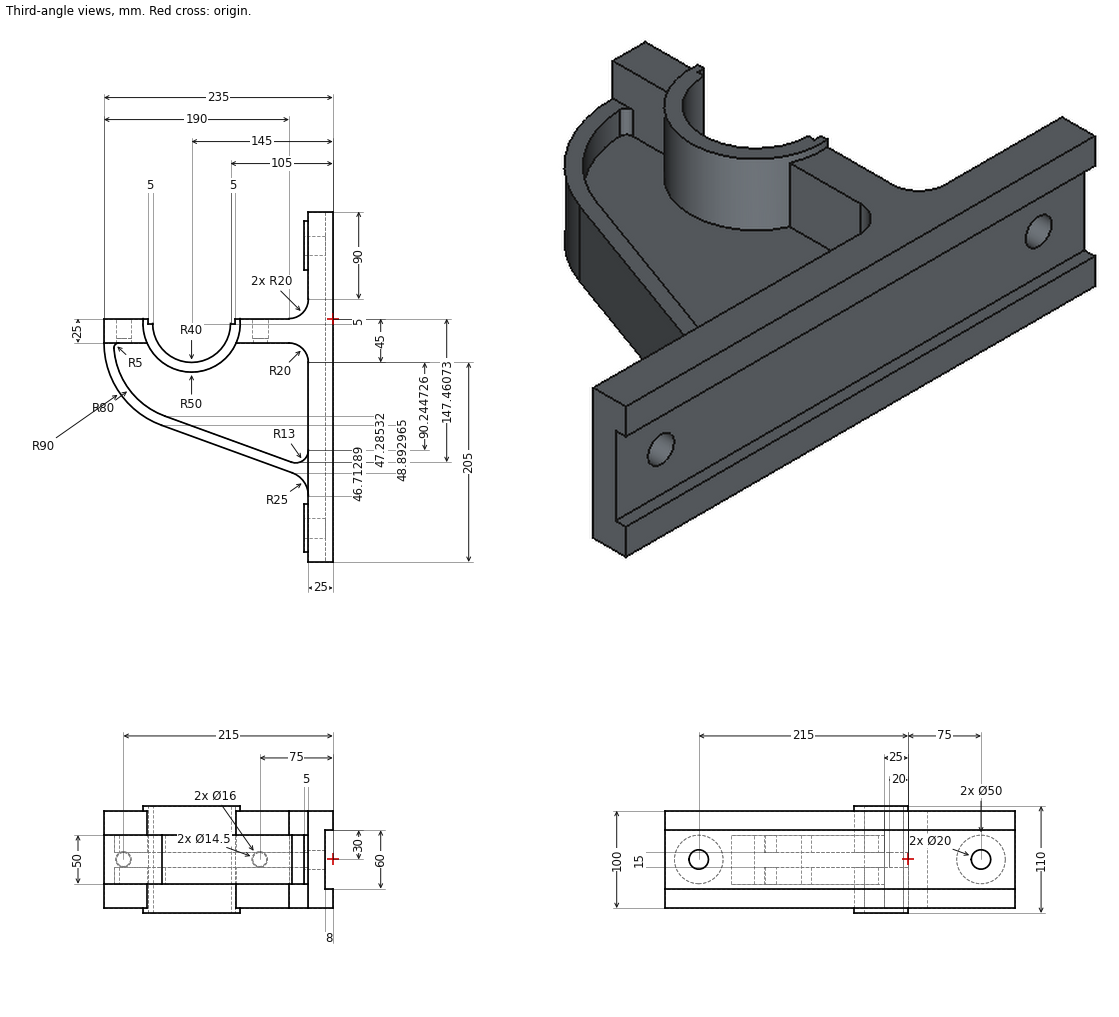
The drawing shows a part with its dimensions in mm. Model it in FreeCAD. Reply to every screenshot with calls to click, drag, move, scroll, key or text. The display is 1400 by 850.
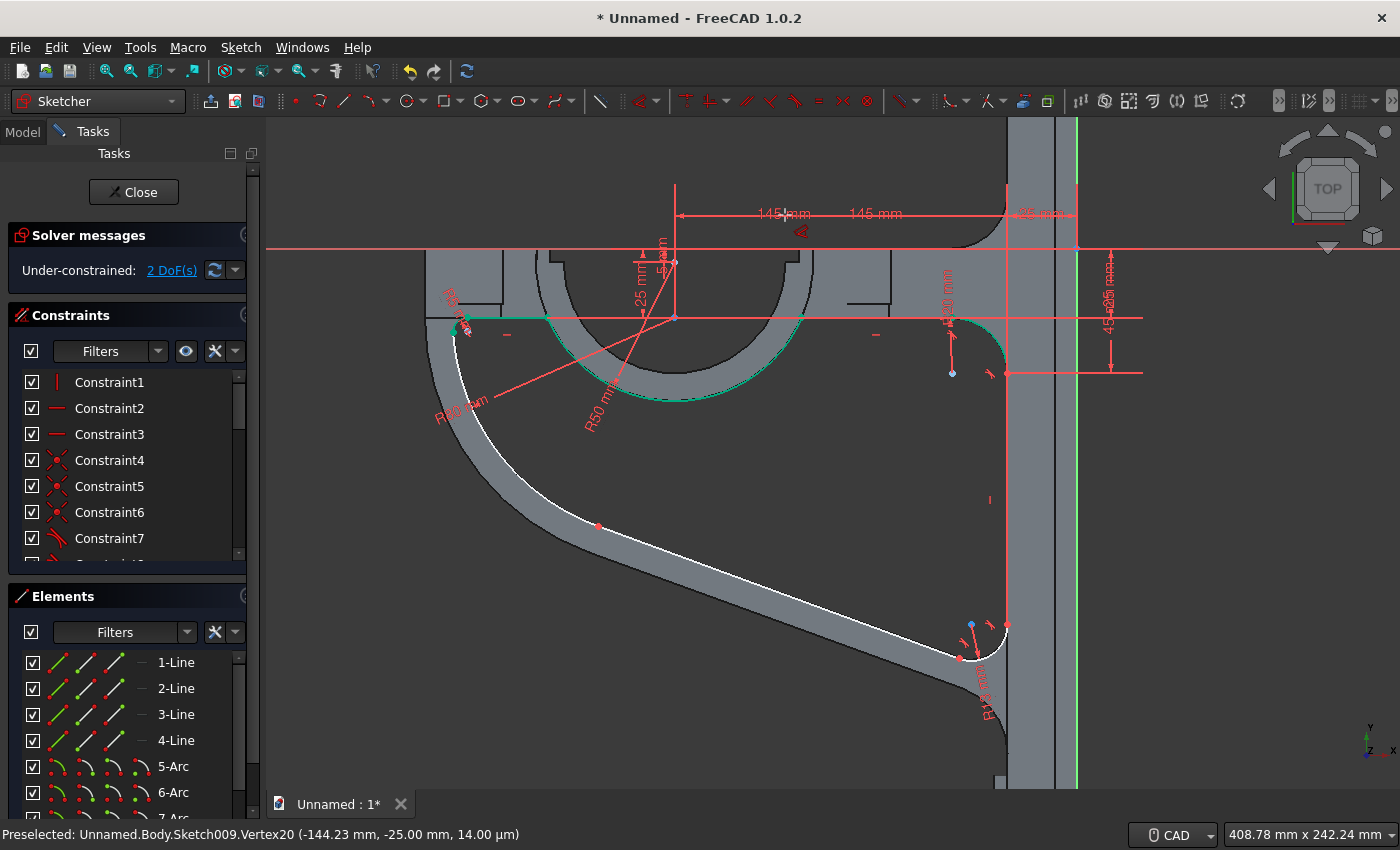
click(1007, 549)
click(1041, 499)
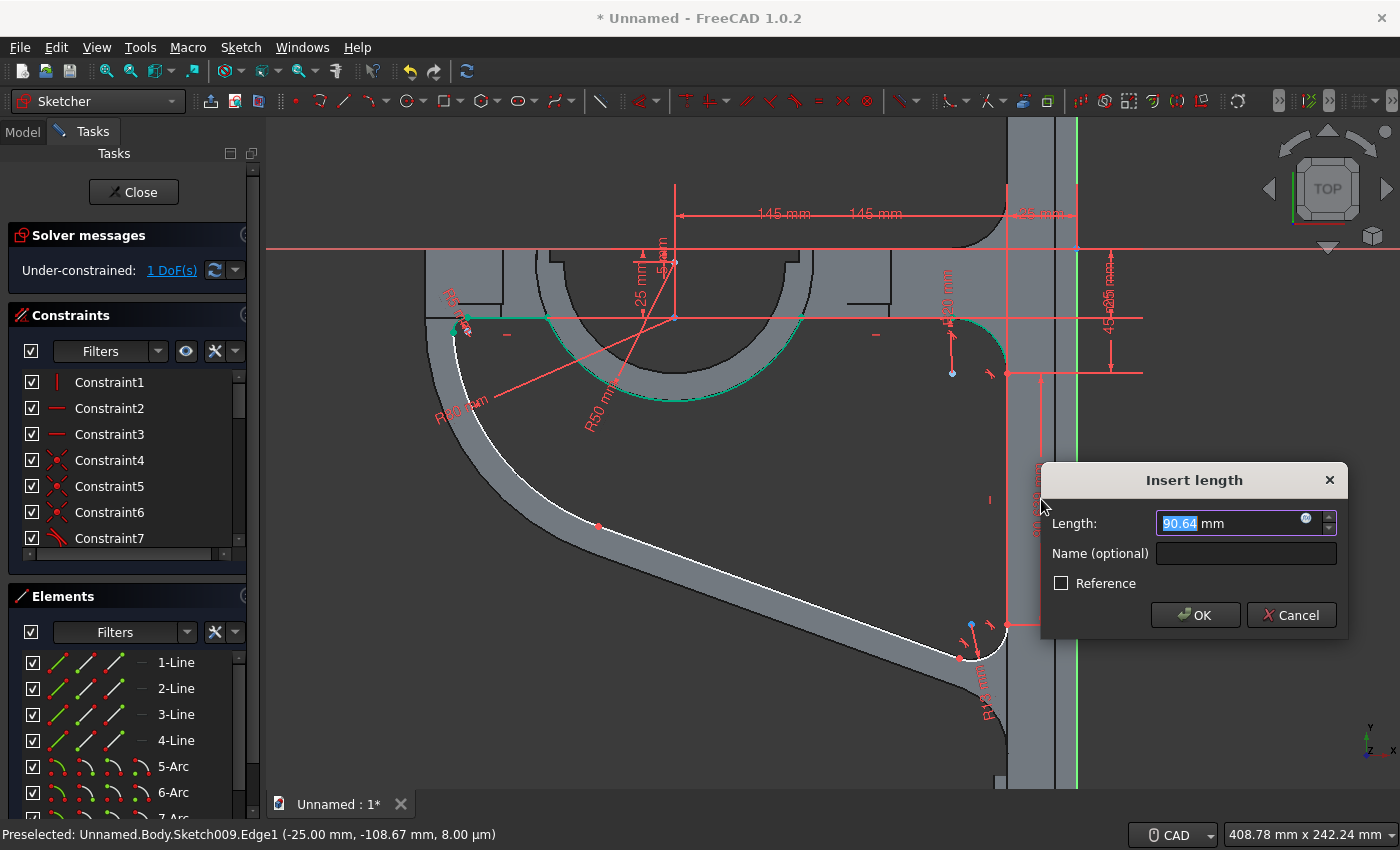
text(90.244726)
key(Return)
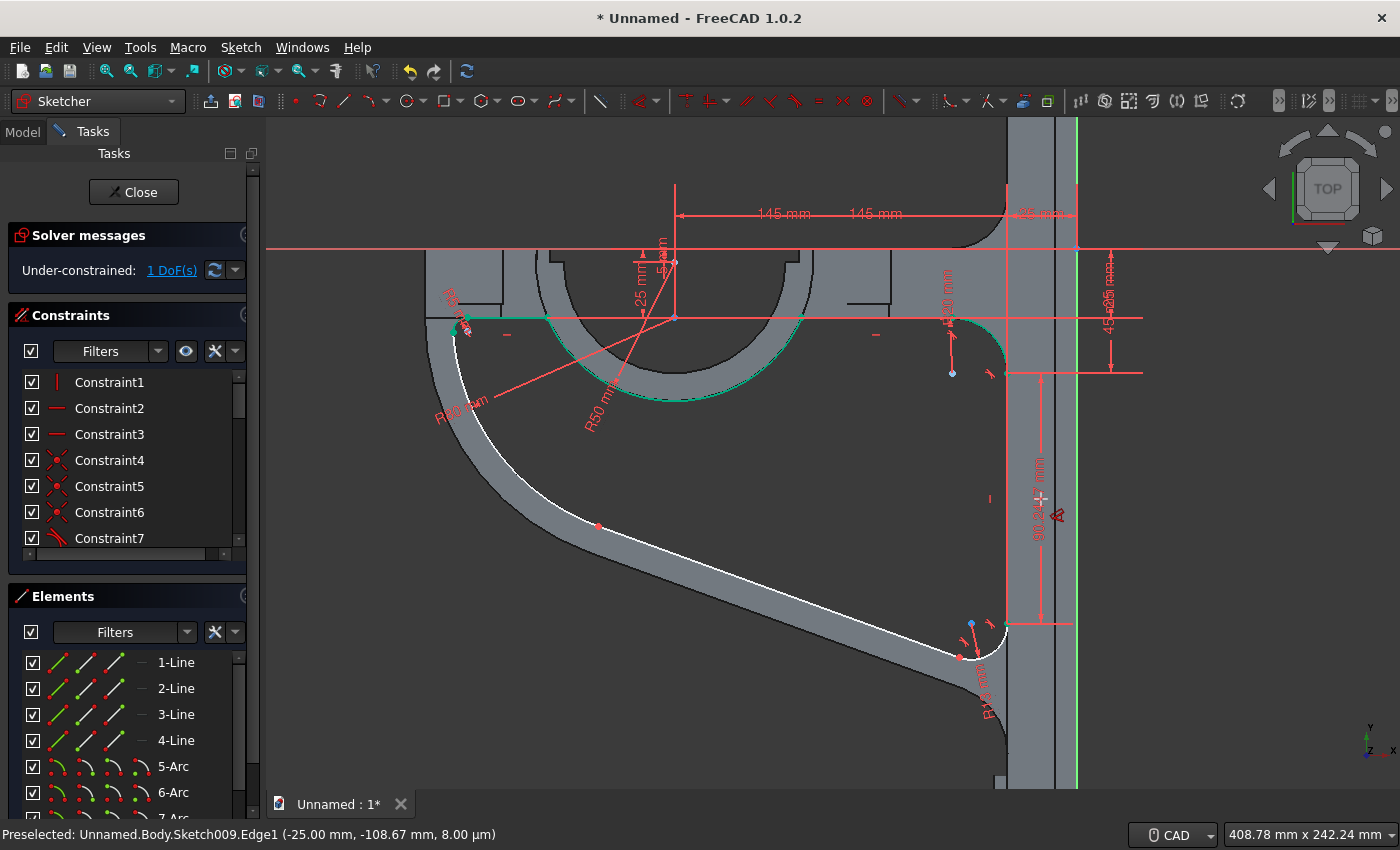
click(707, 566)
click(993, 592)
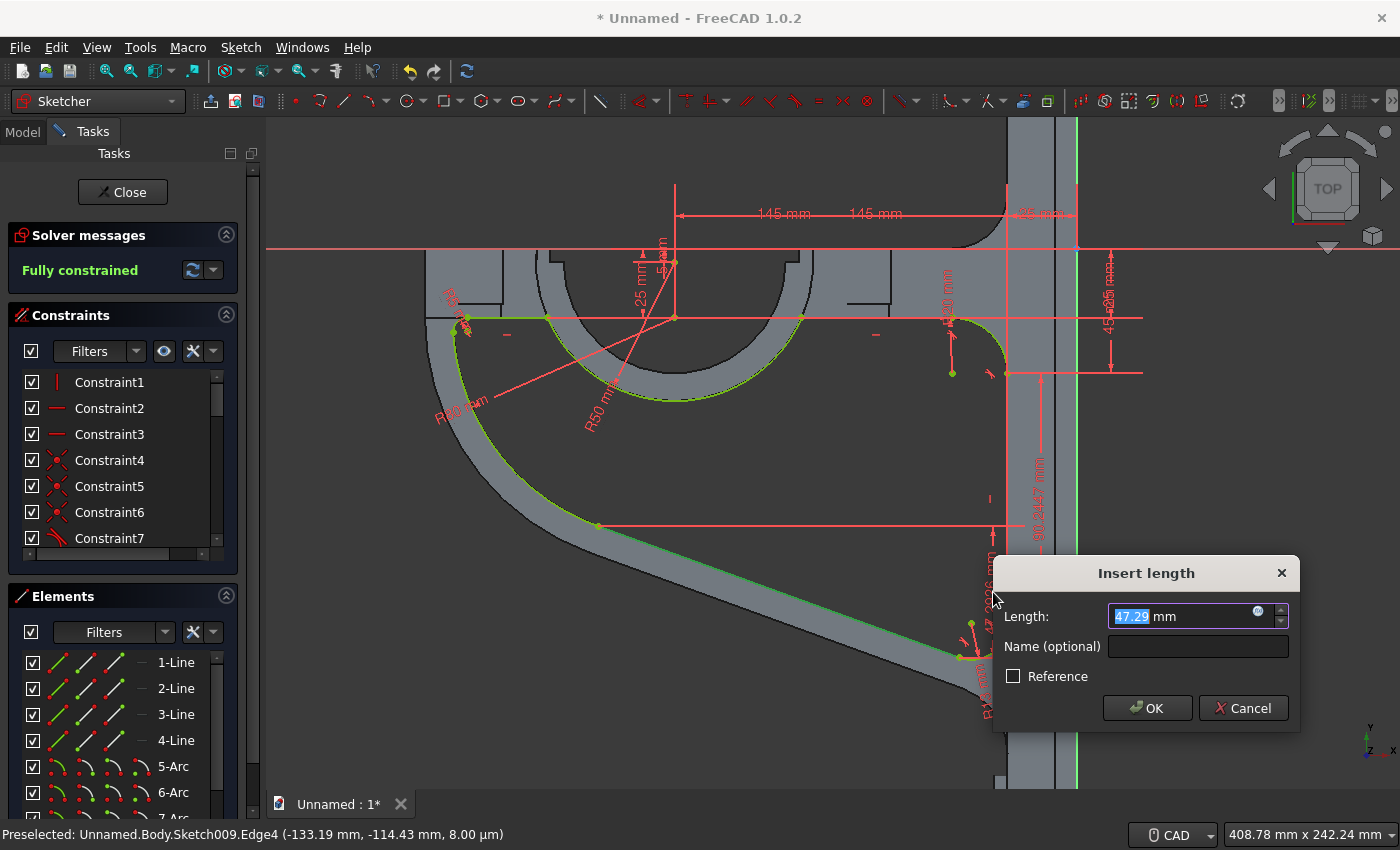
text(47.28532)
key(Return)
key(Escape)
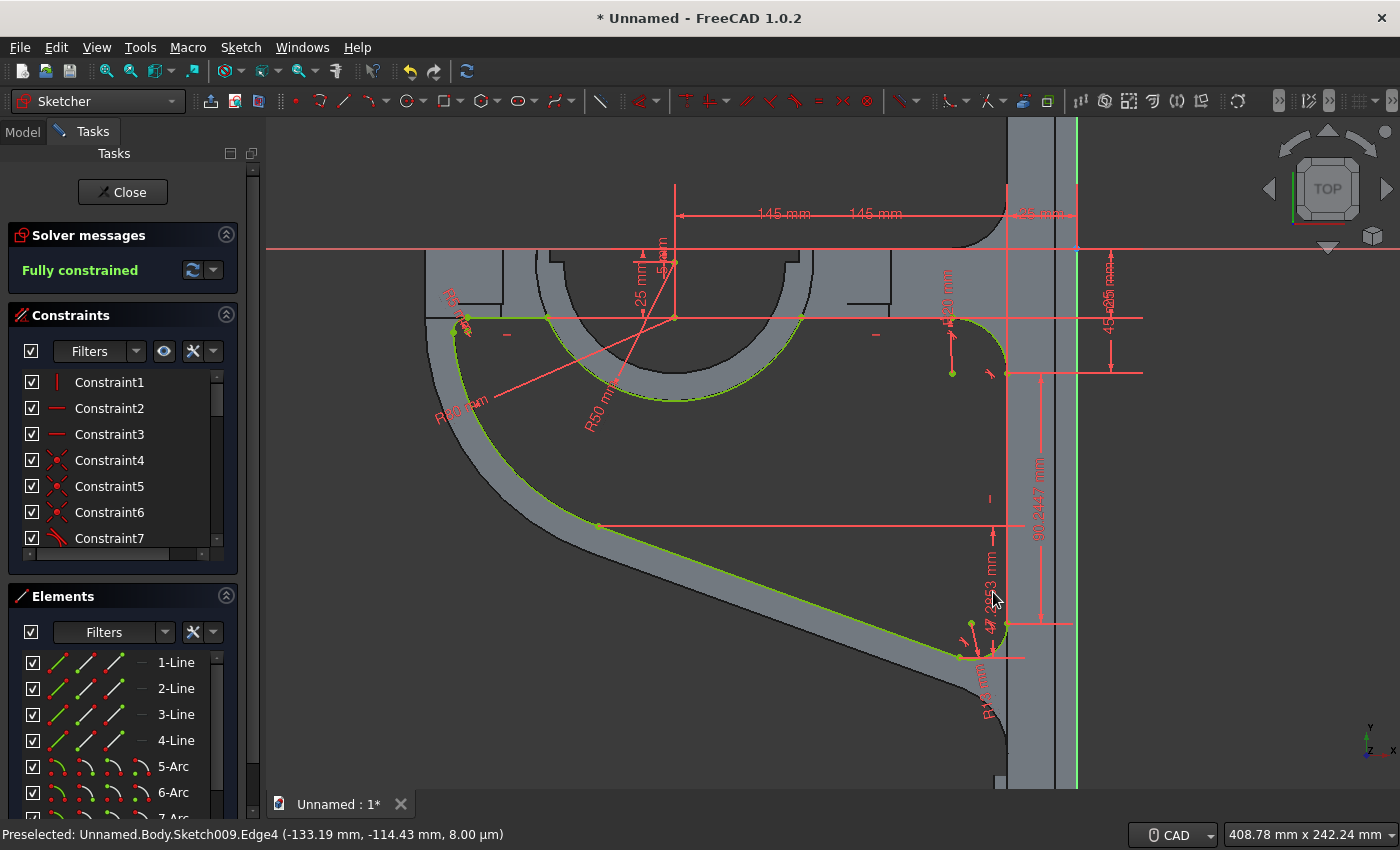
click(123, 192)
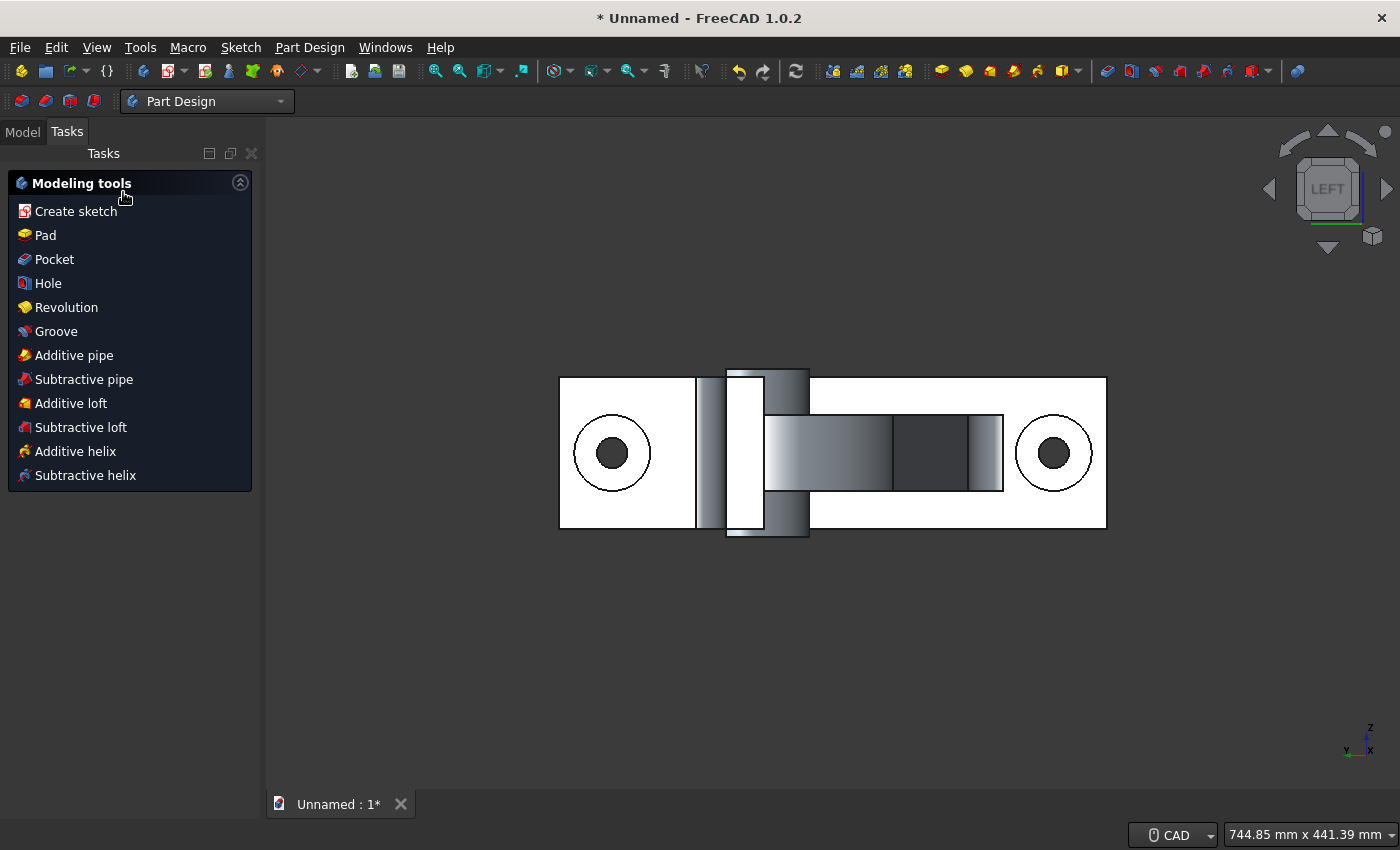
click(942, 72)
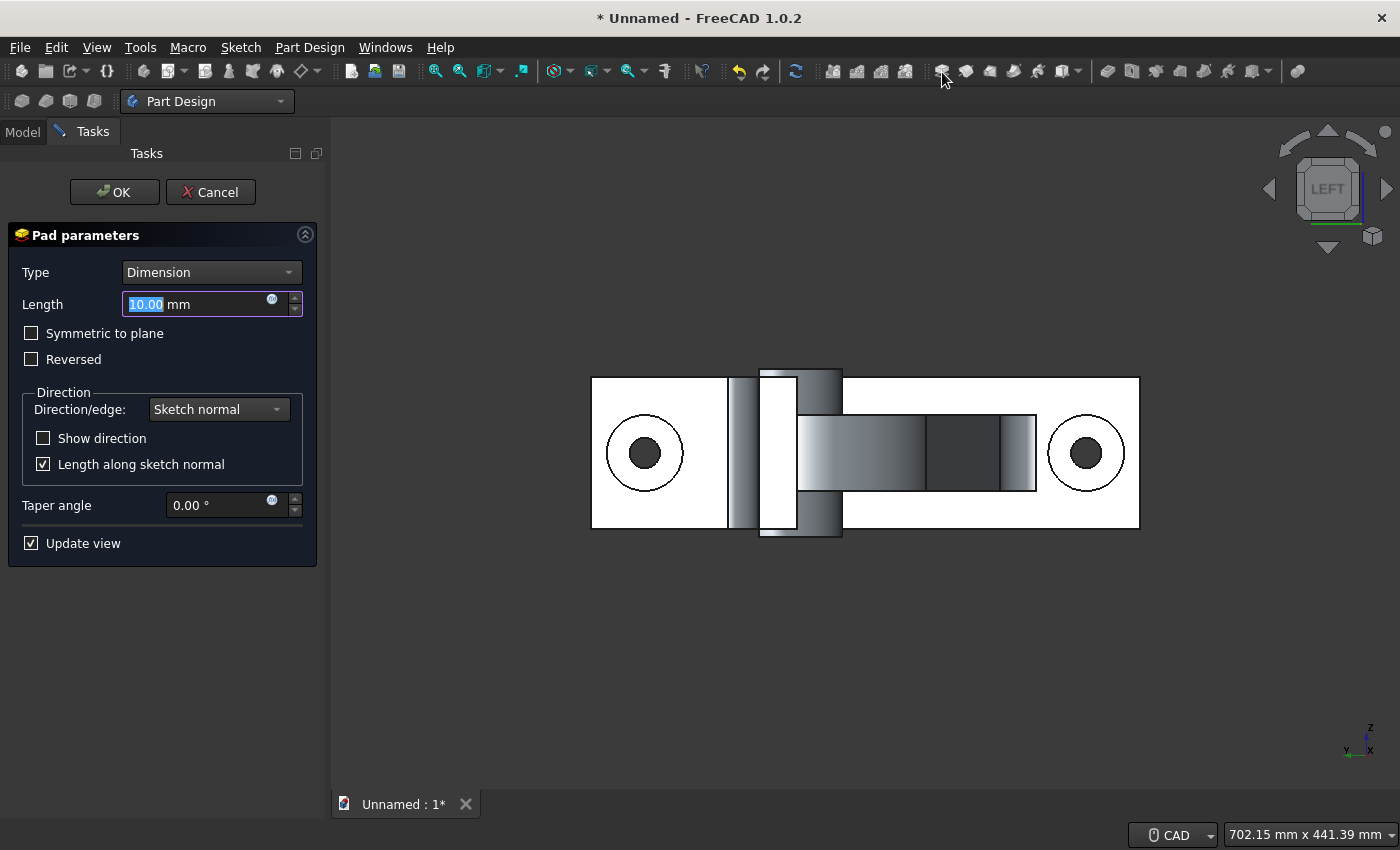
text(15)
key(Tab)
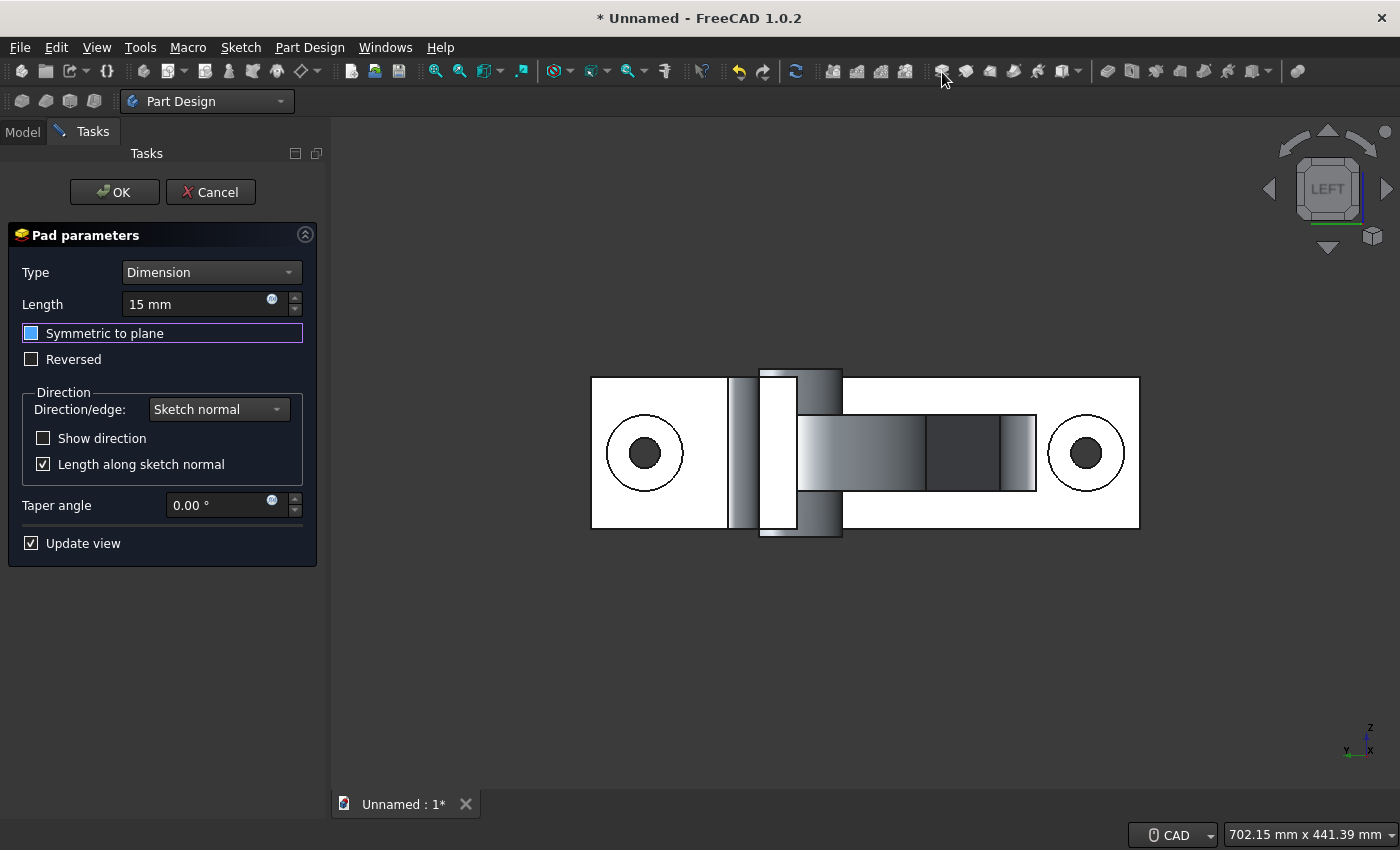
click(30, 333)